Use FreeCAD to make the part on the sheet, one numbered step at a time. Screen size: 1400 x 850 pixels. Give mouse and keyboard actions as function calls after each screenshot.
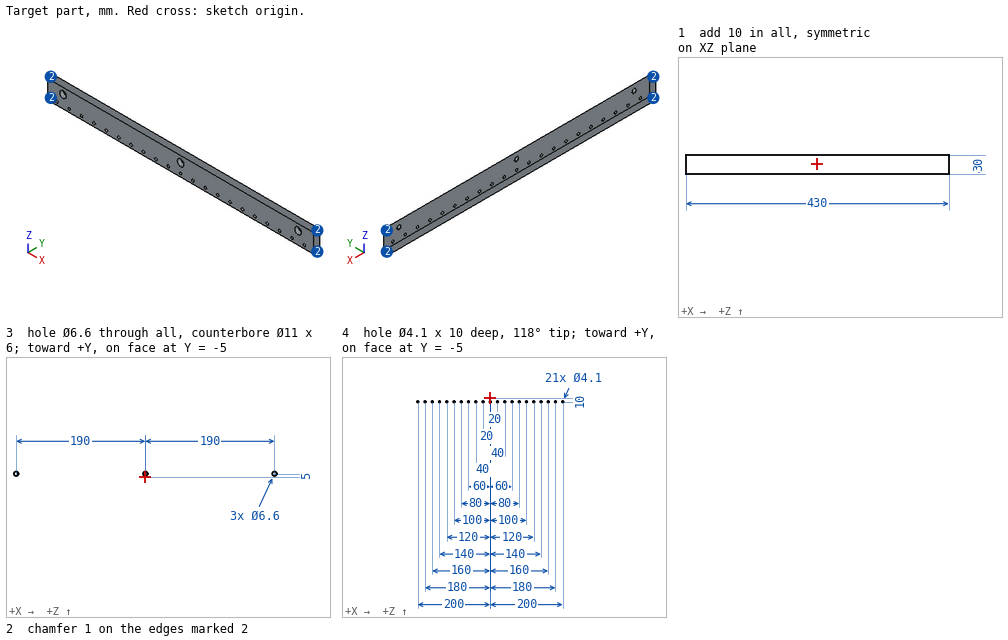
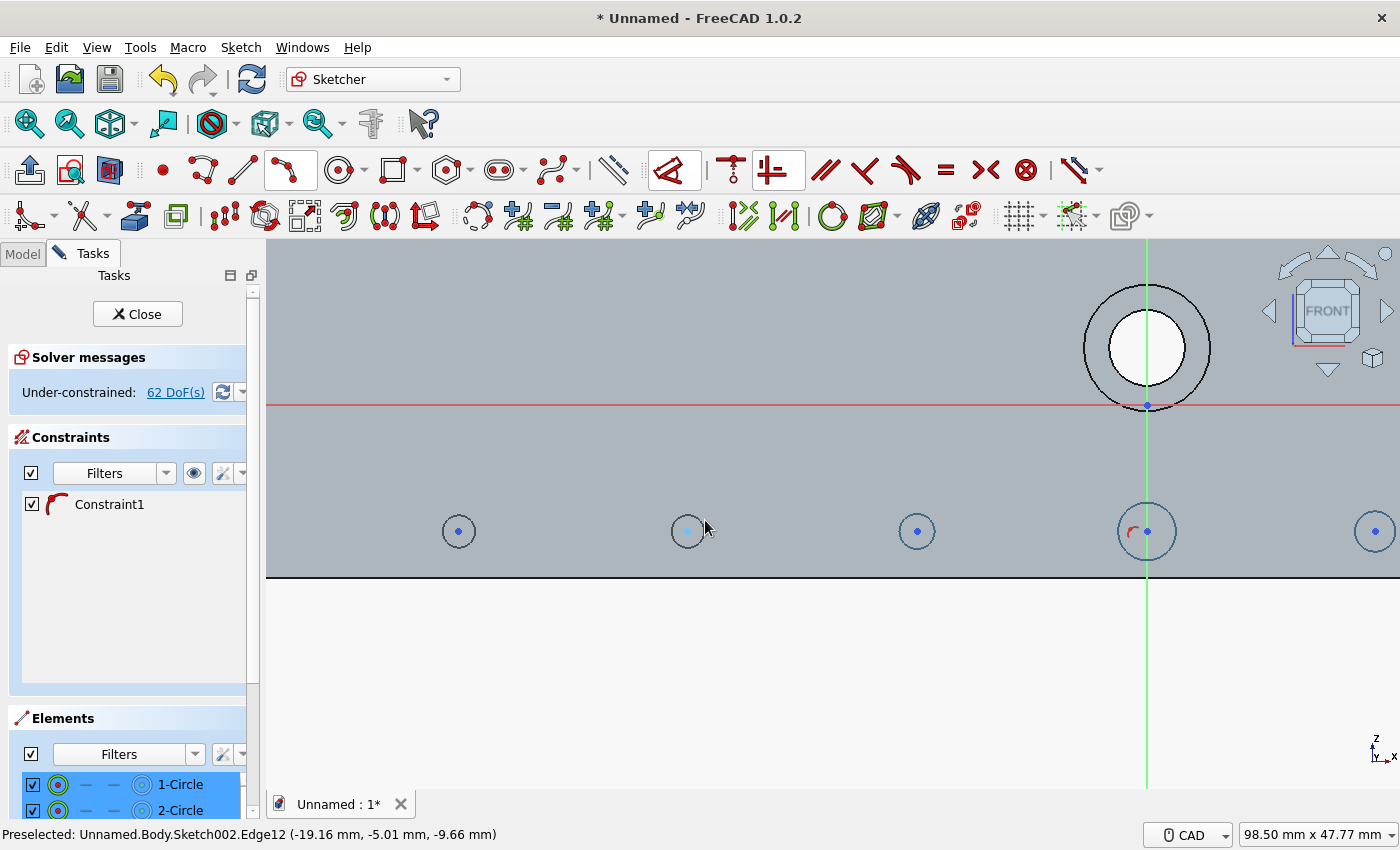
click(699, 520)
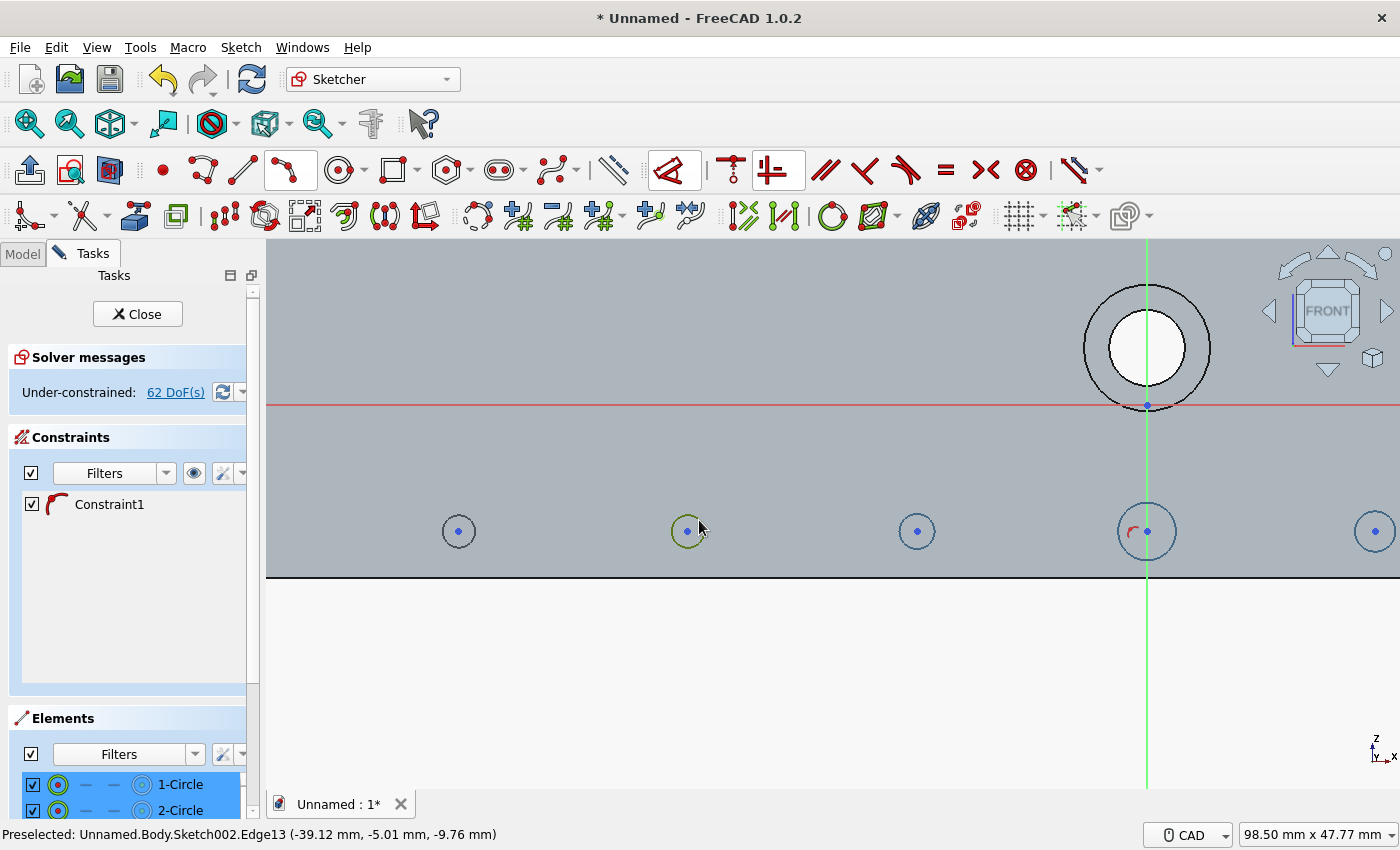
click(470, 520)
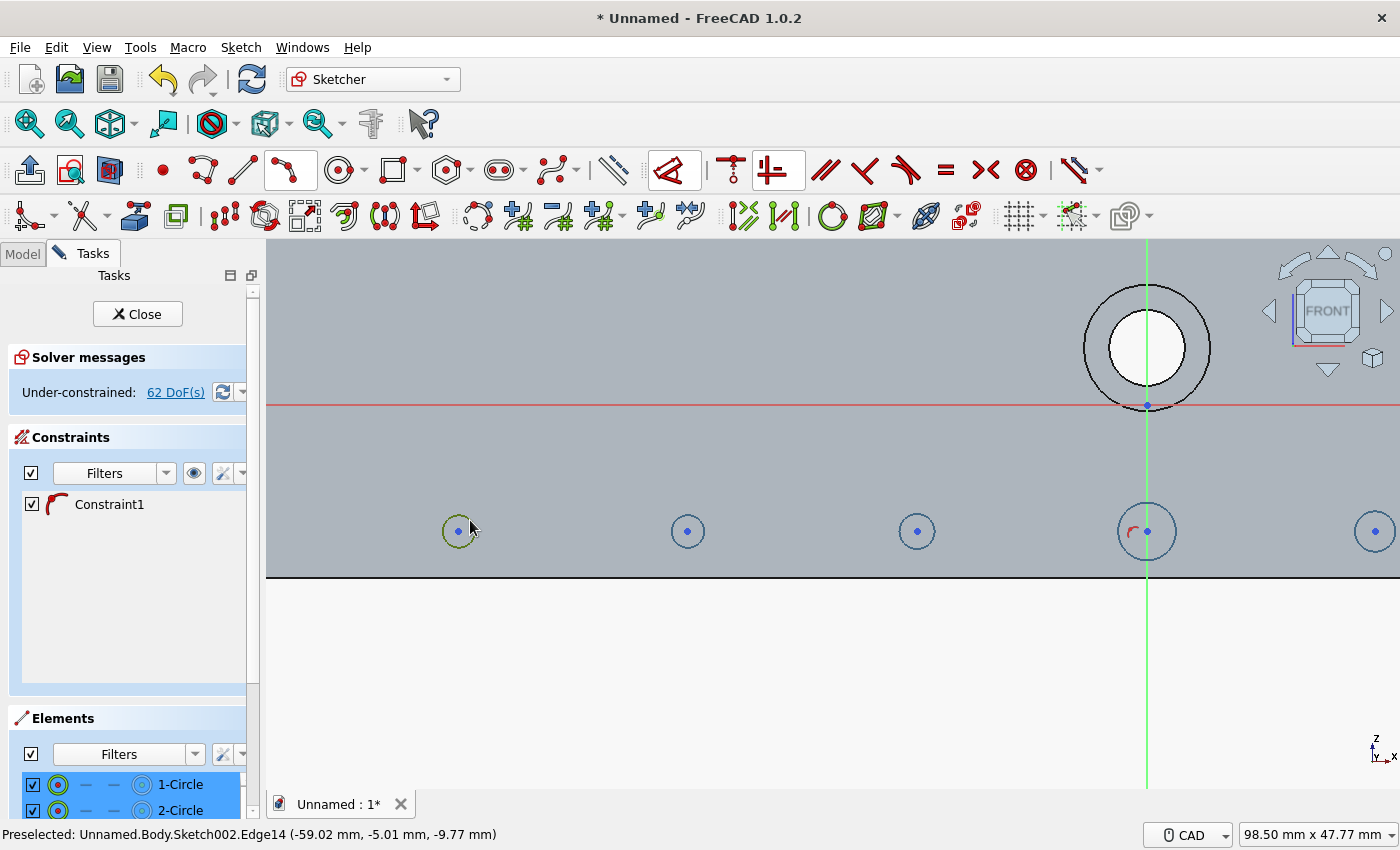
scroll(705, 520, down, 10)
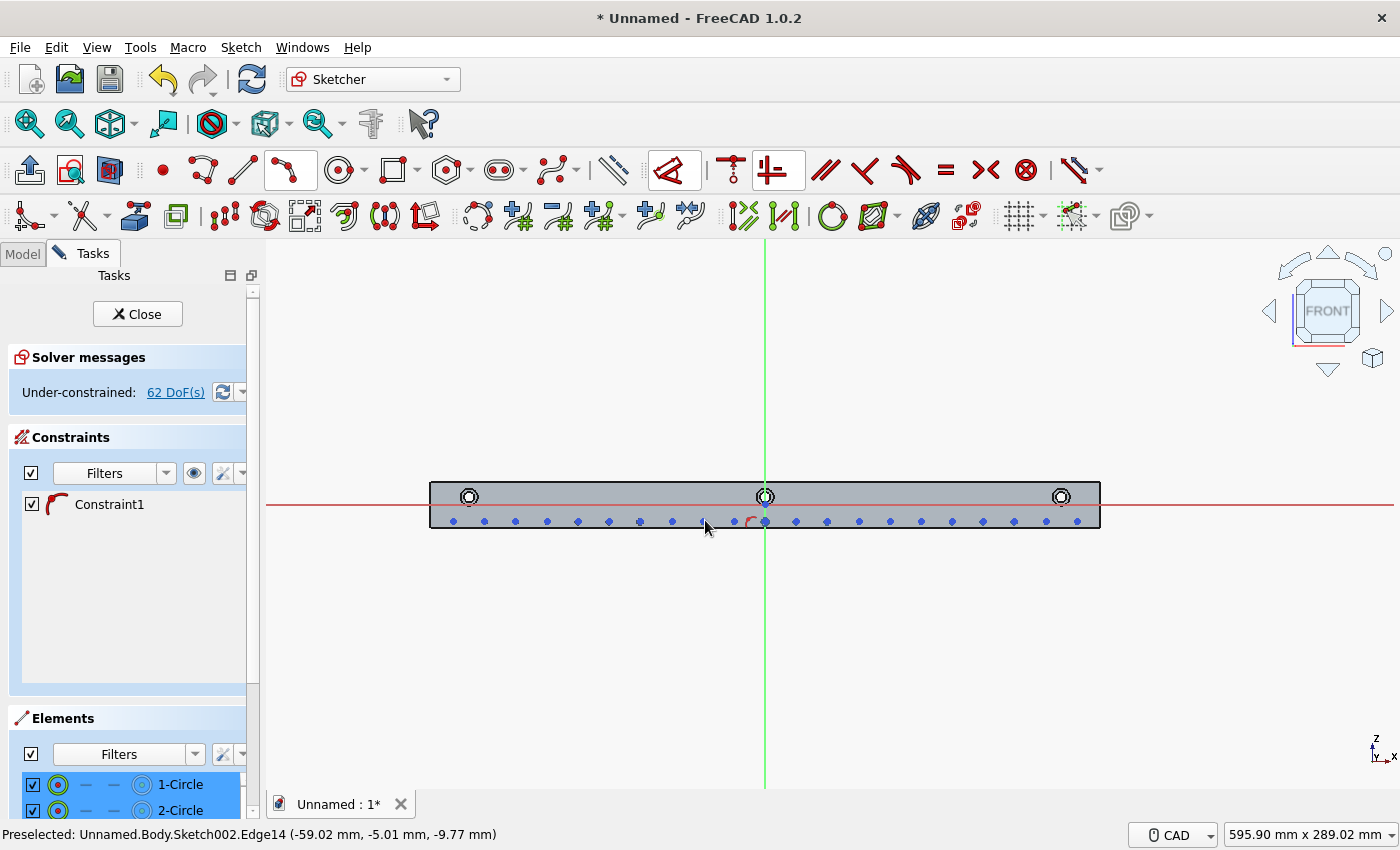
scroll(642, 520, up, 8)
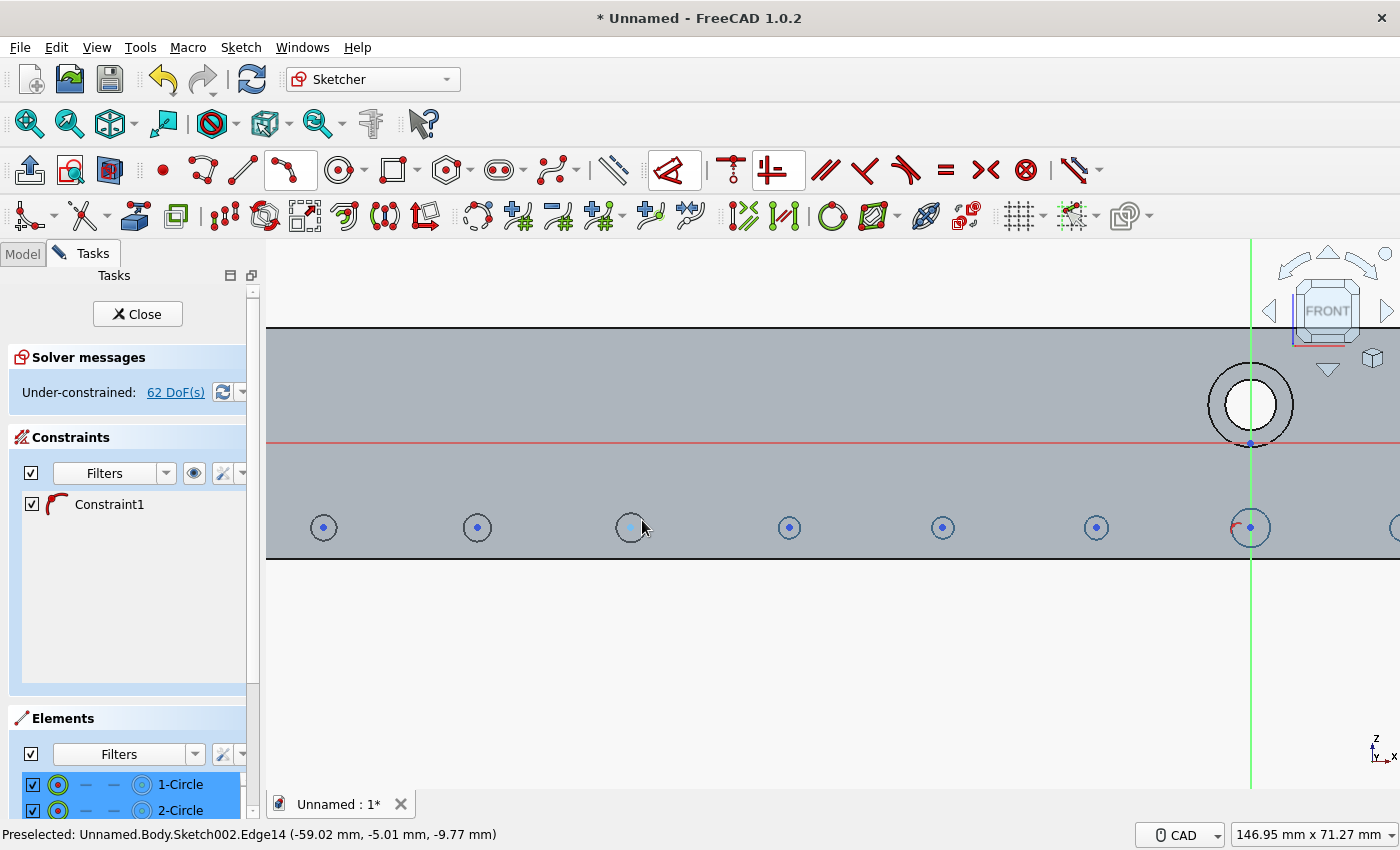
click(641, 518)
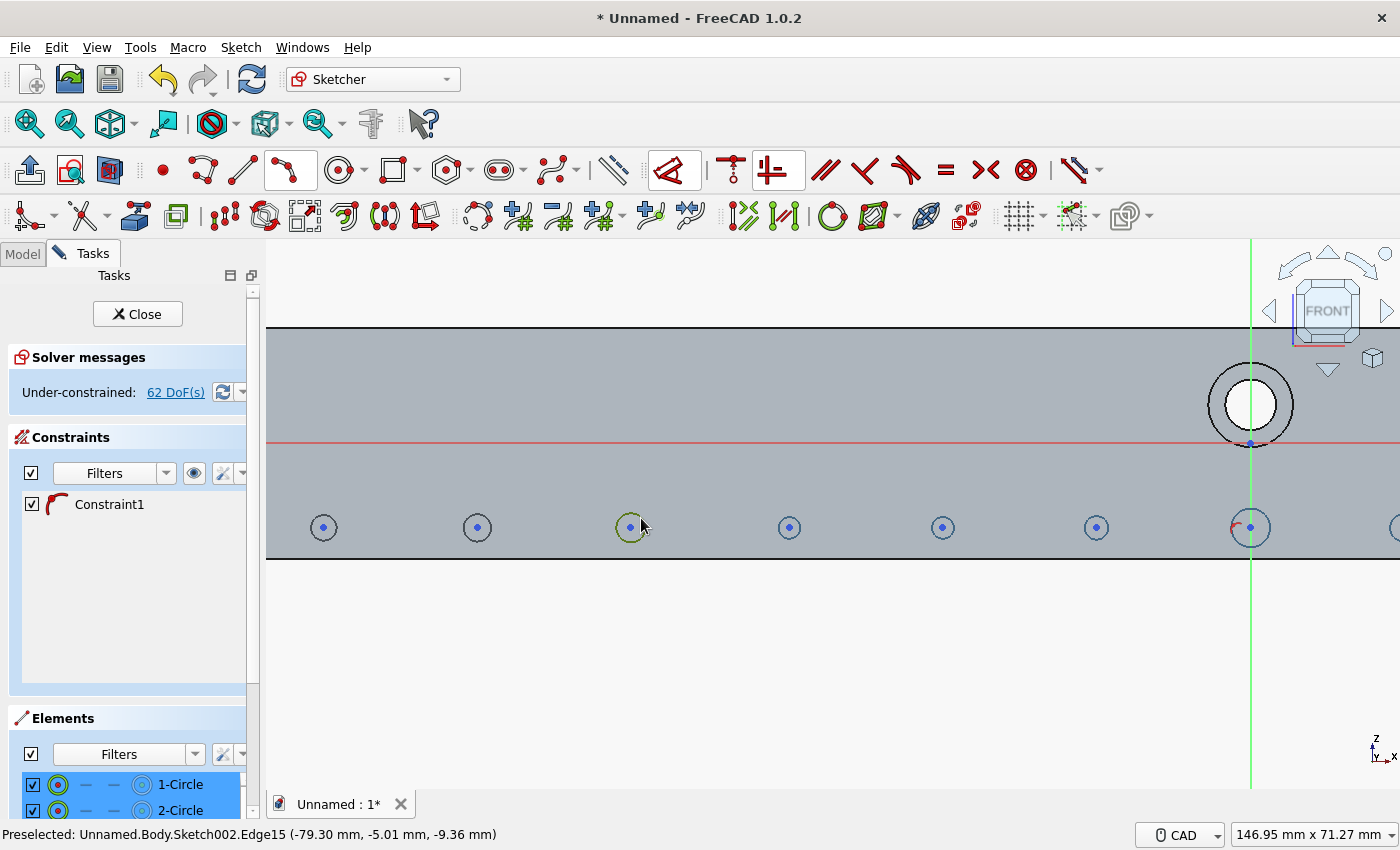
click(487, 518)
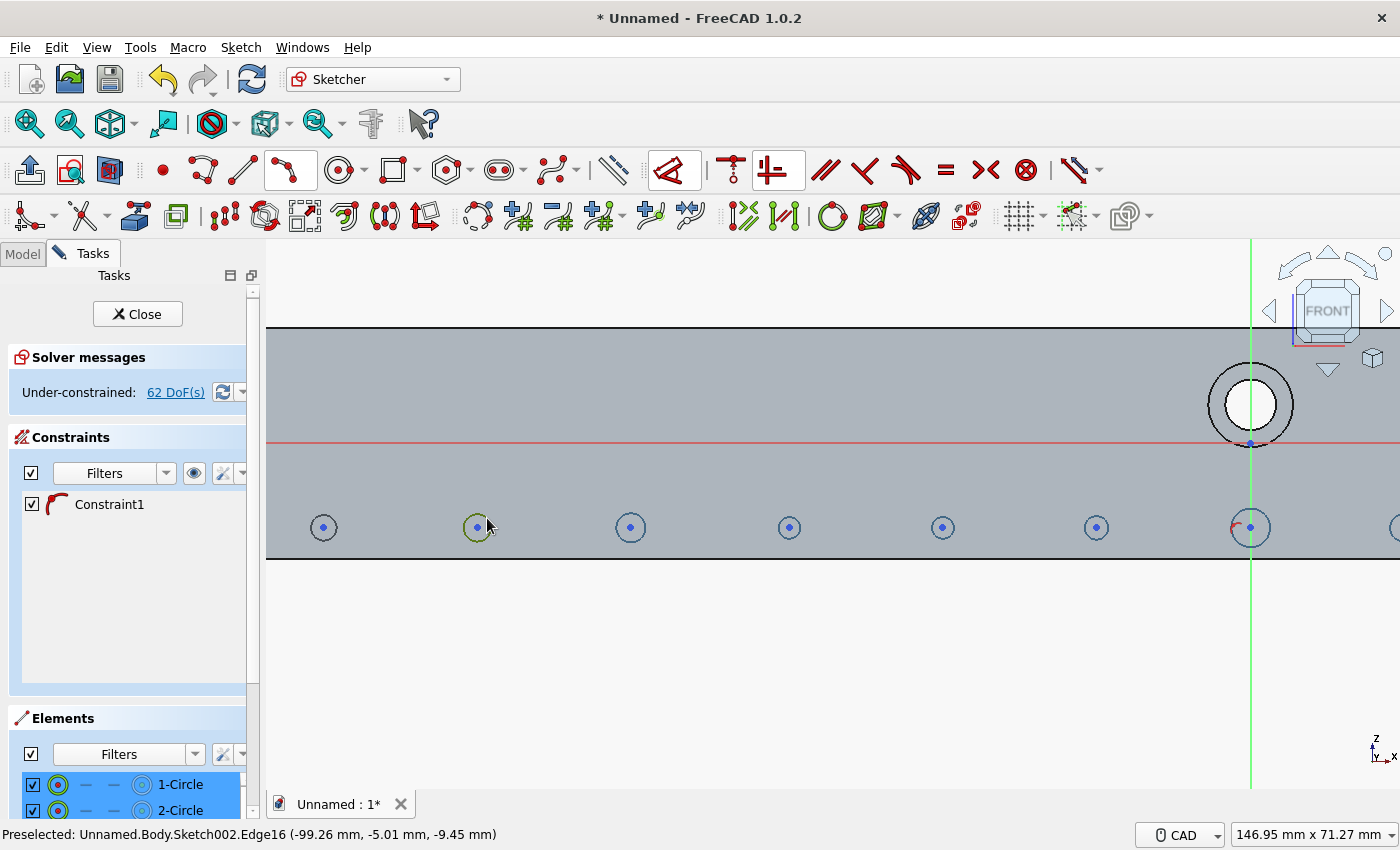
click(333, 519)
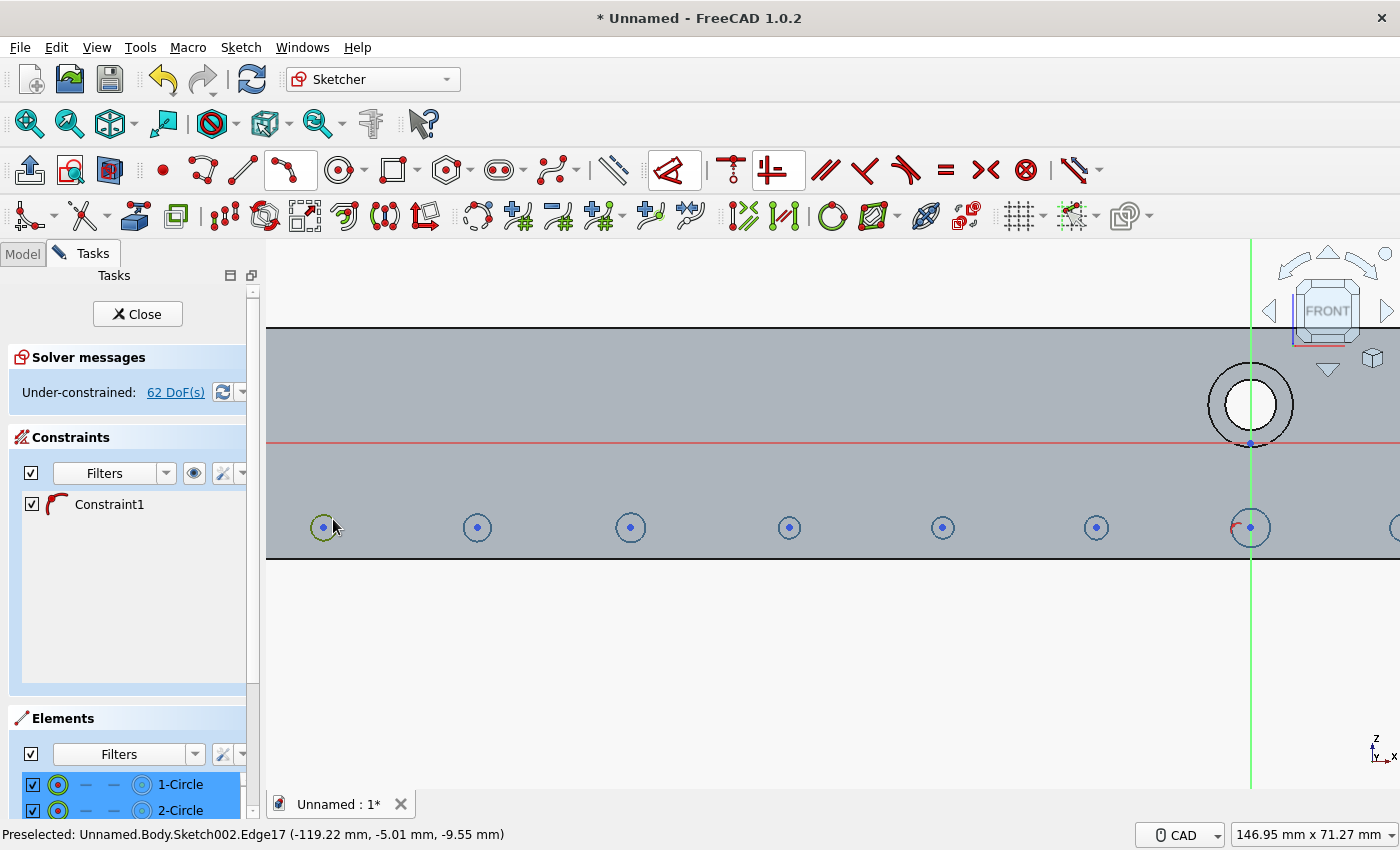
scroll(642, 520, down, 8)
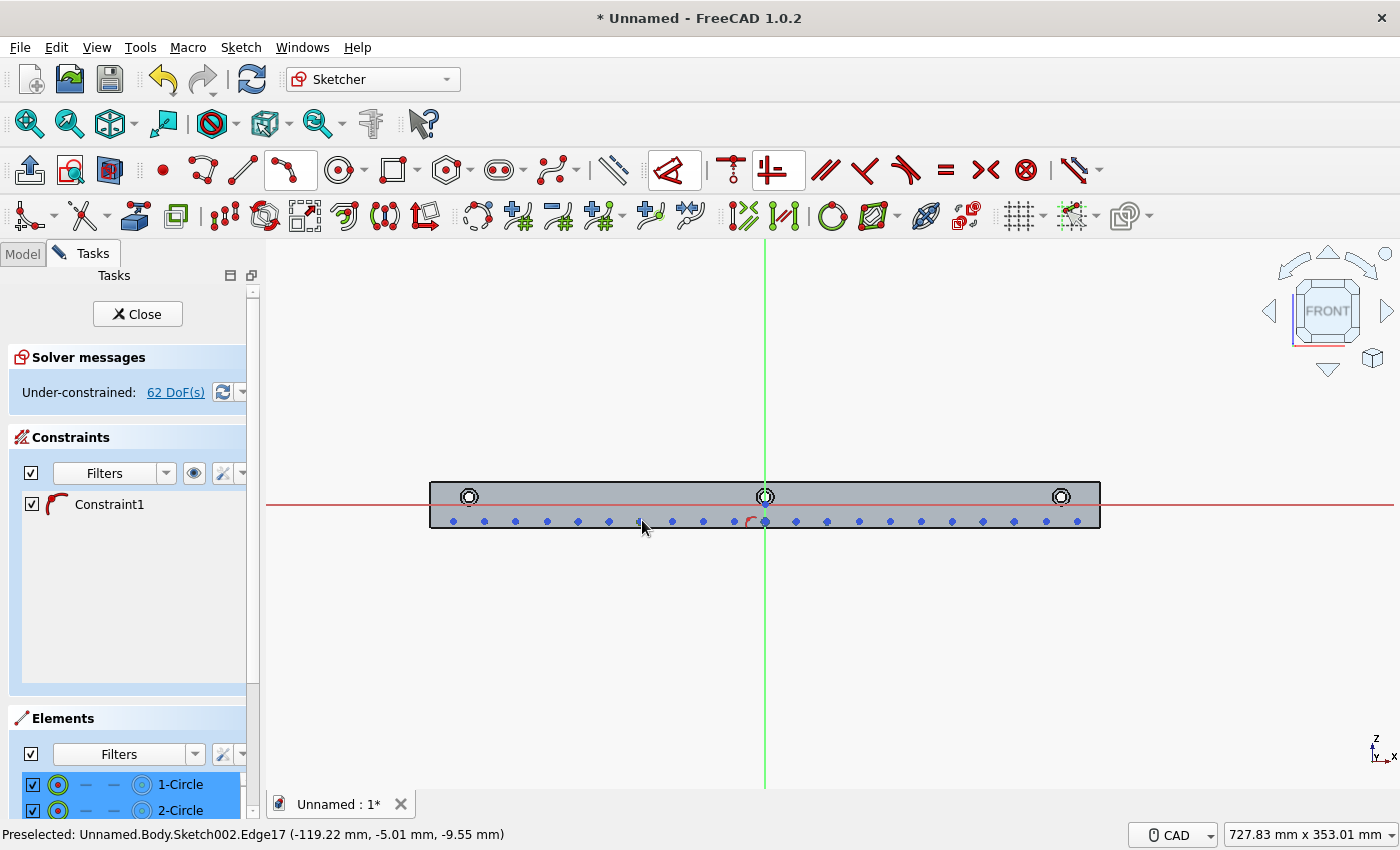
scroll(549, 520, up, 9)